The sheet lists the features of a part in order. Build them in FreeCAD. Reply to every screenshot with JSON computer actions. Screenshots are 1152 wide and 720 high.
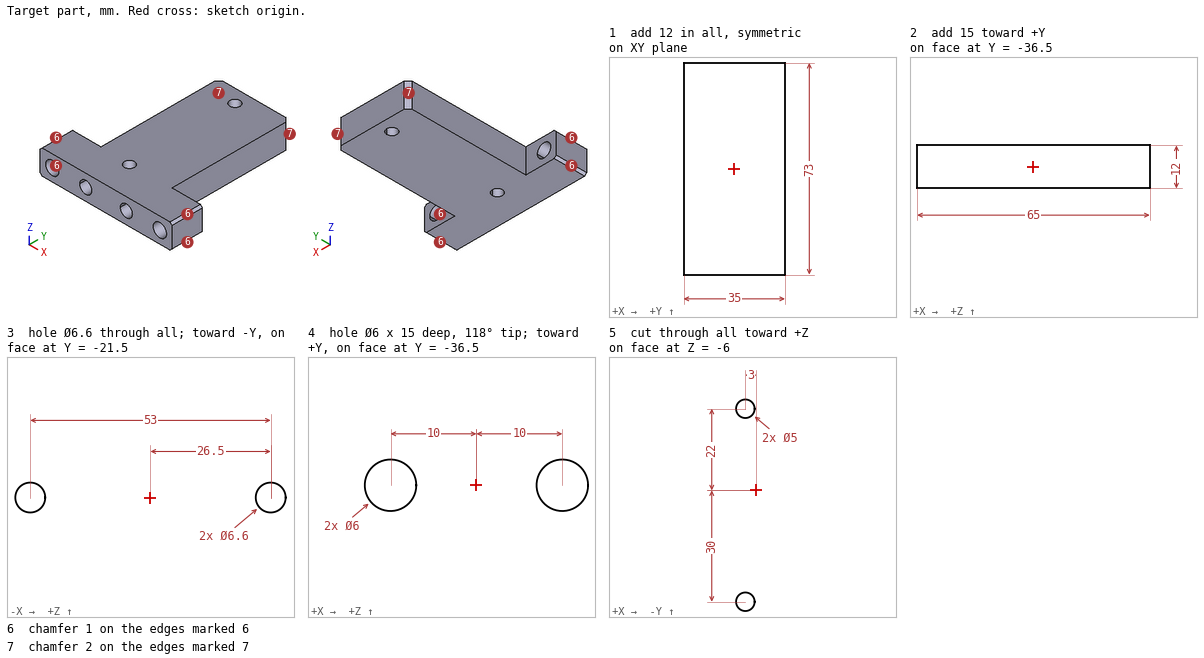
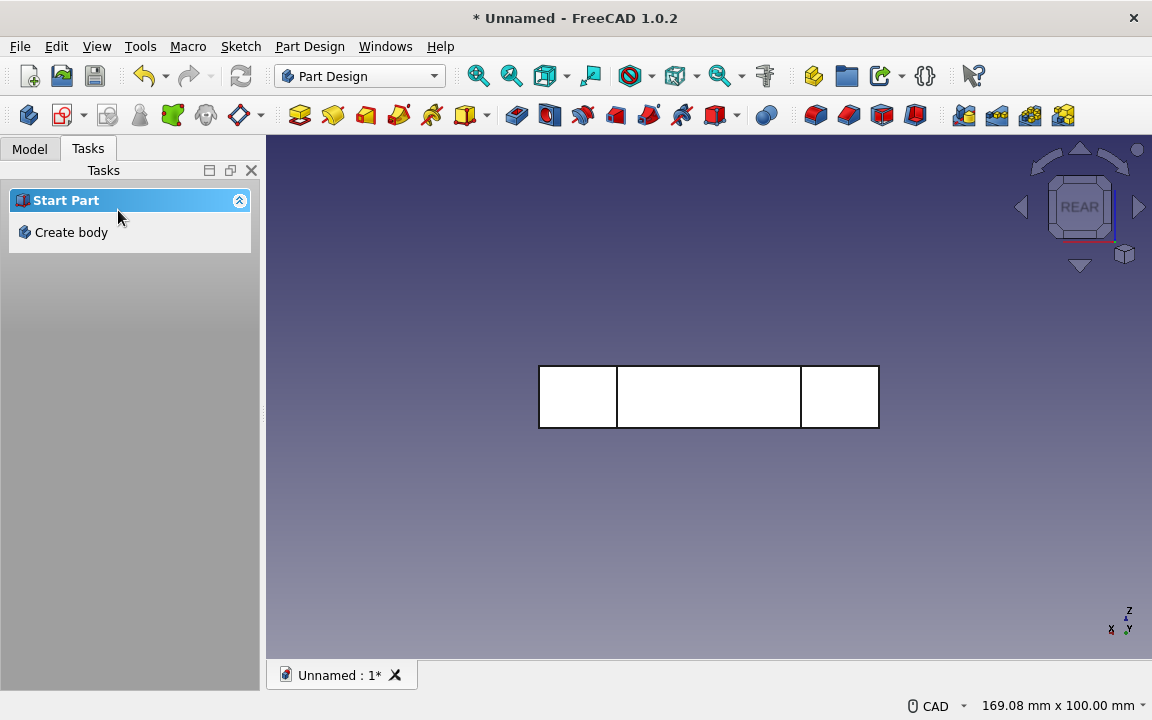
{"action": "left_click", "coordinate": [479, 76]}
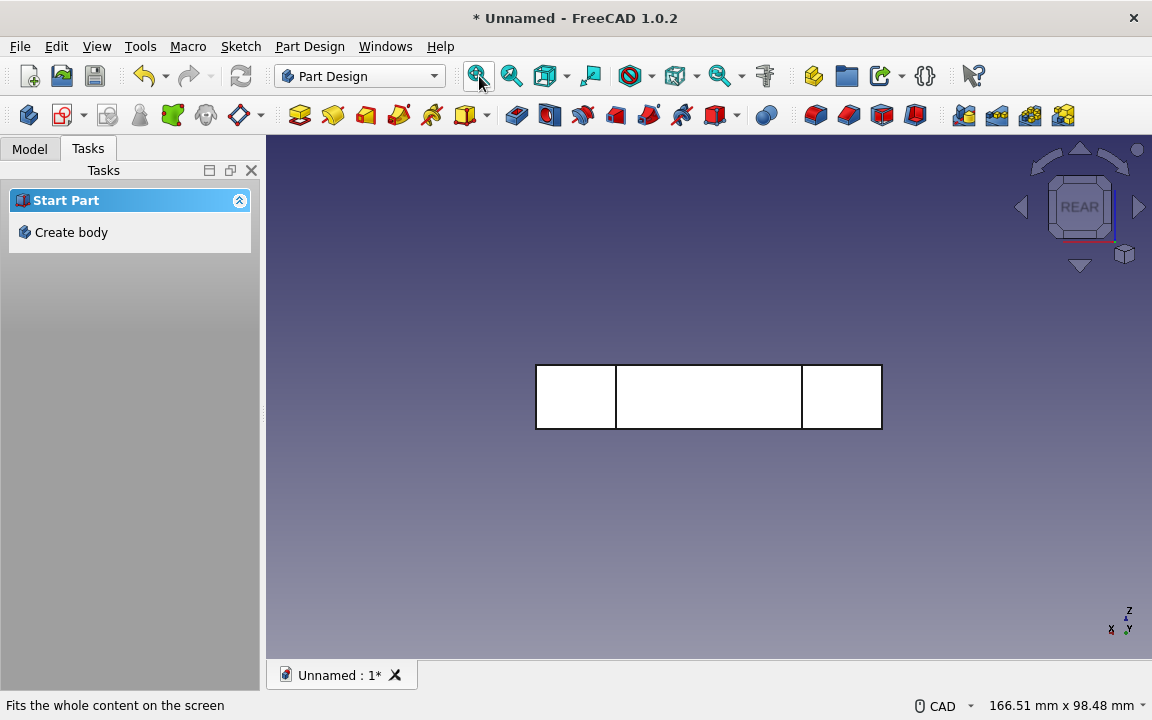
{"action": "left_click", "coordinate": [576, 396]}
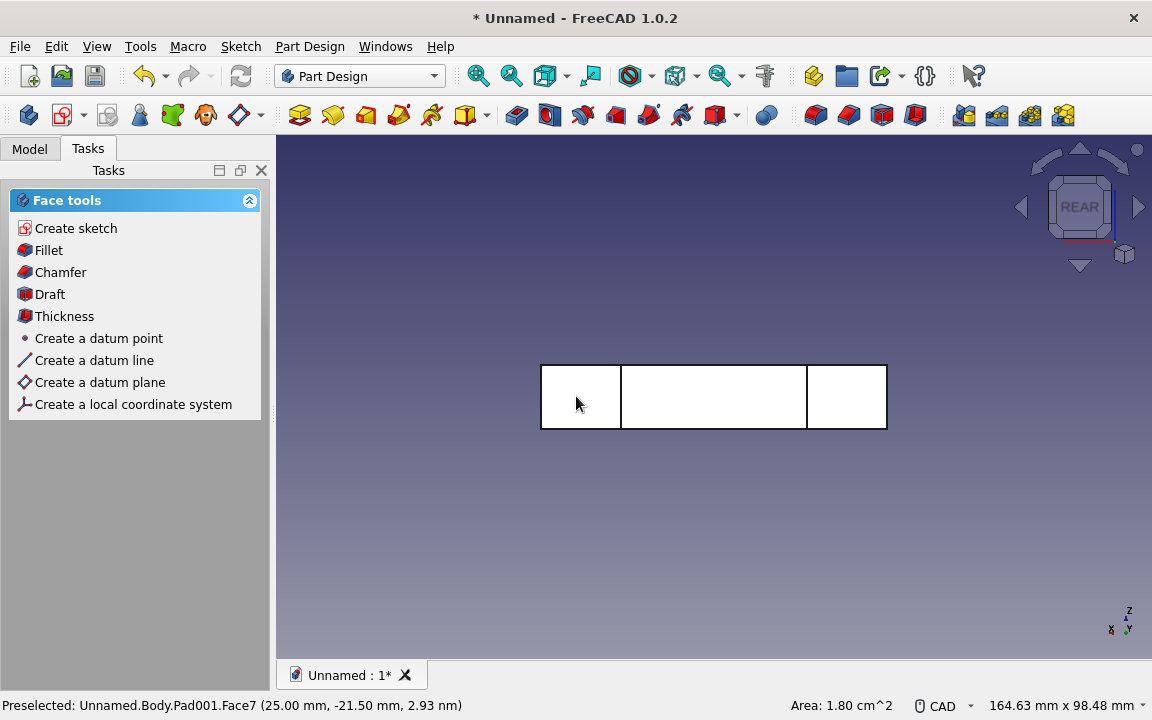
{"action": "left_click", "coordinate": [62, 116]}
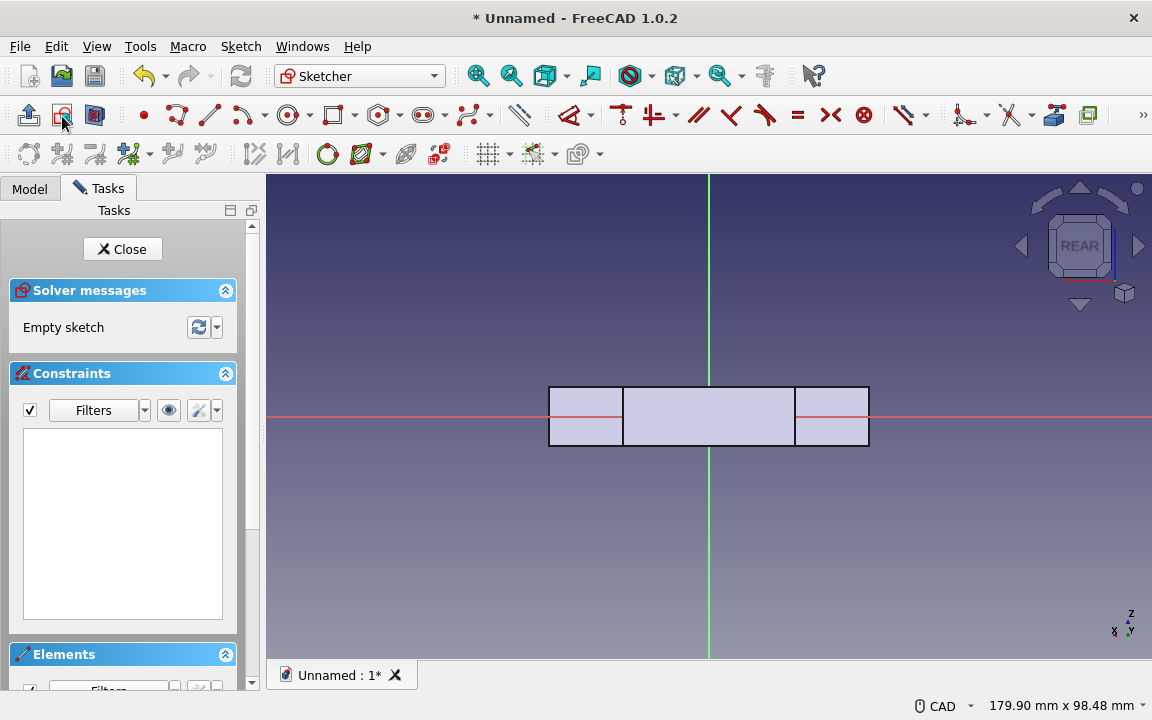
{"action": "scroll", "coordinate": [792, 417], "scroll_direction": "up", "scroll_amount": 3}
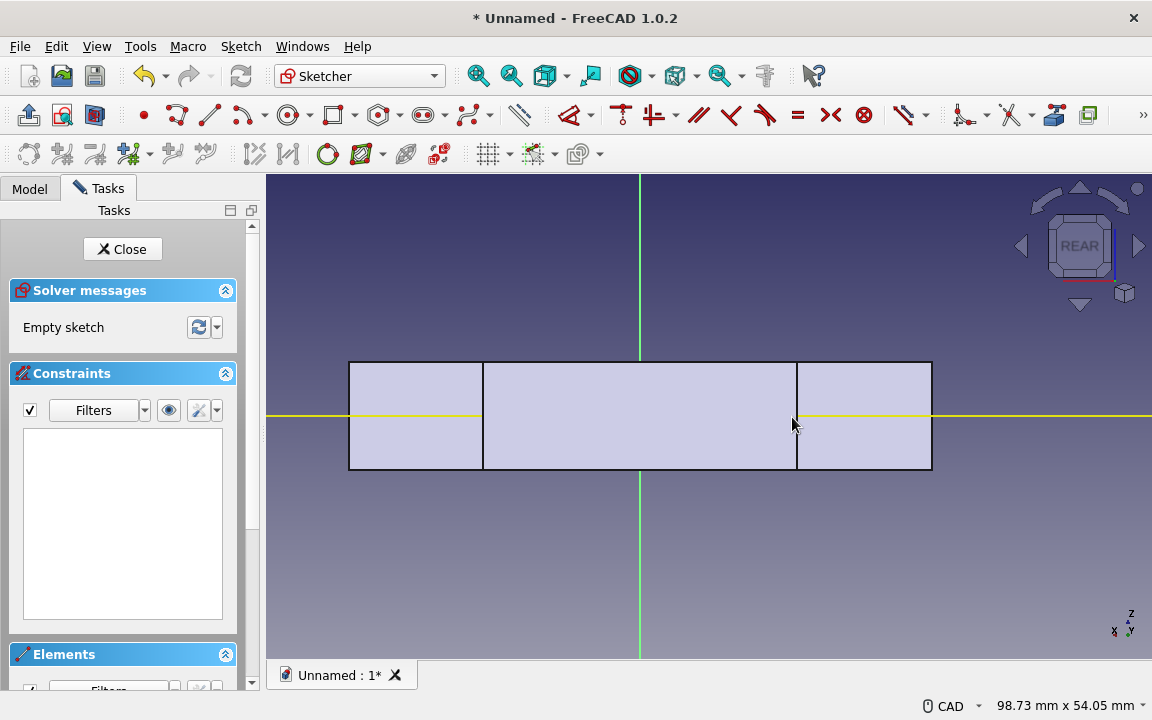
{"action": "left_click", "coordinate": [288, 116]}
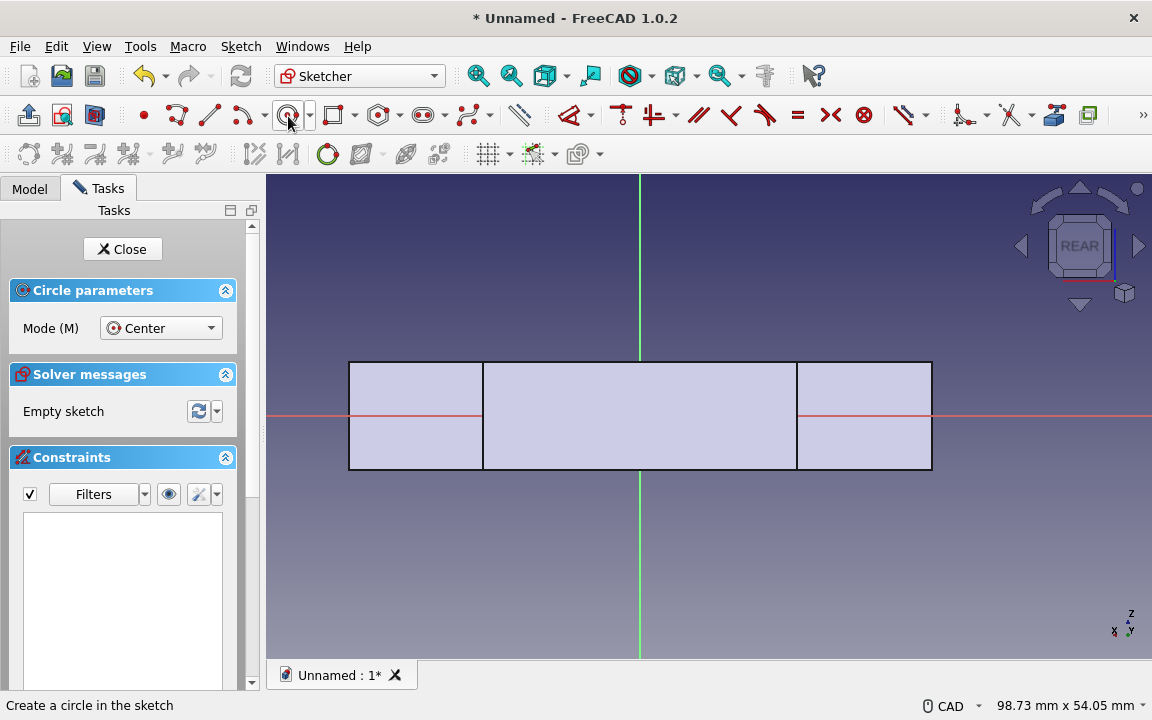
{"action": "left_click", "coordinate": [878, 416]}
{"action": "mouse_move", "coordinate": [899, 395]}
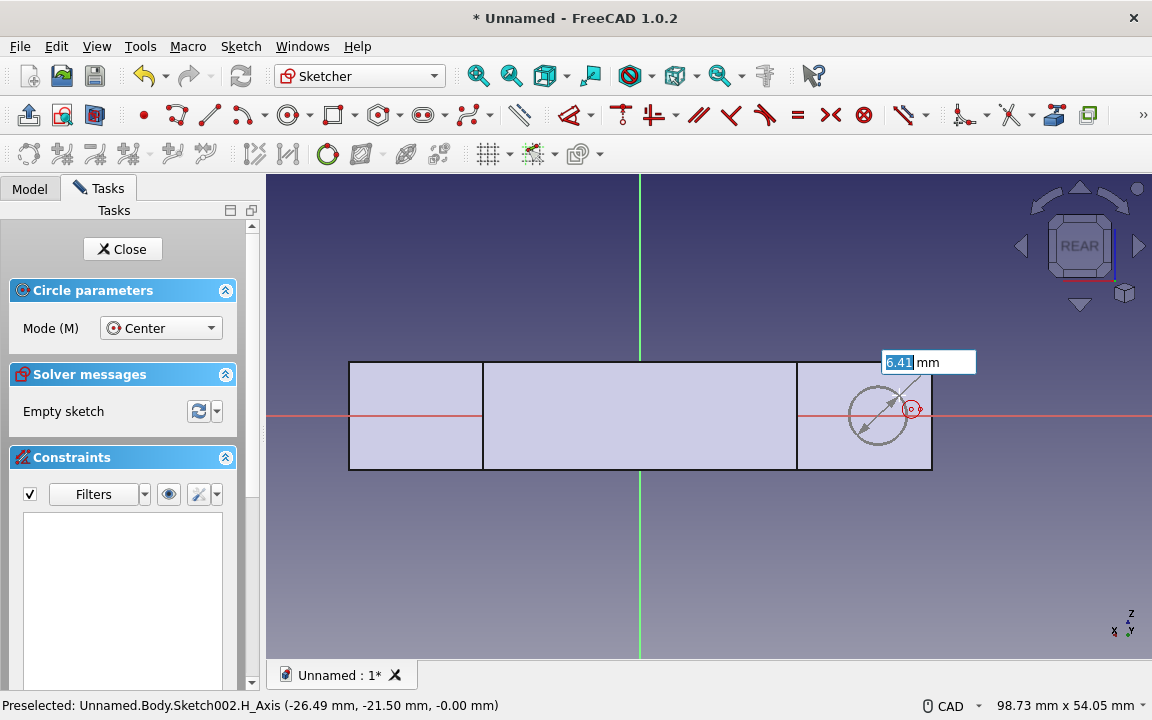
{"action": "type", "text": "6.6"}
{"action": "key", "text": "Return"}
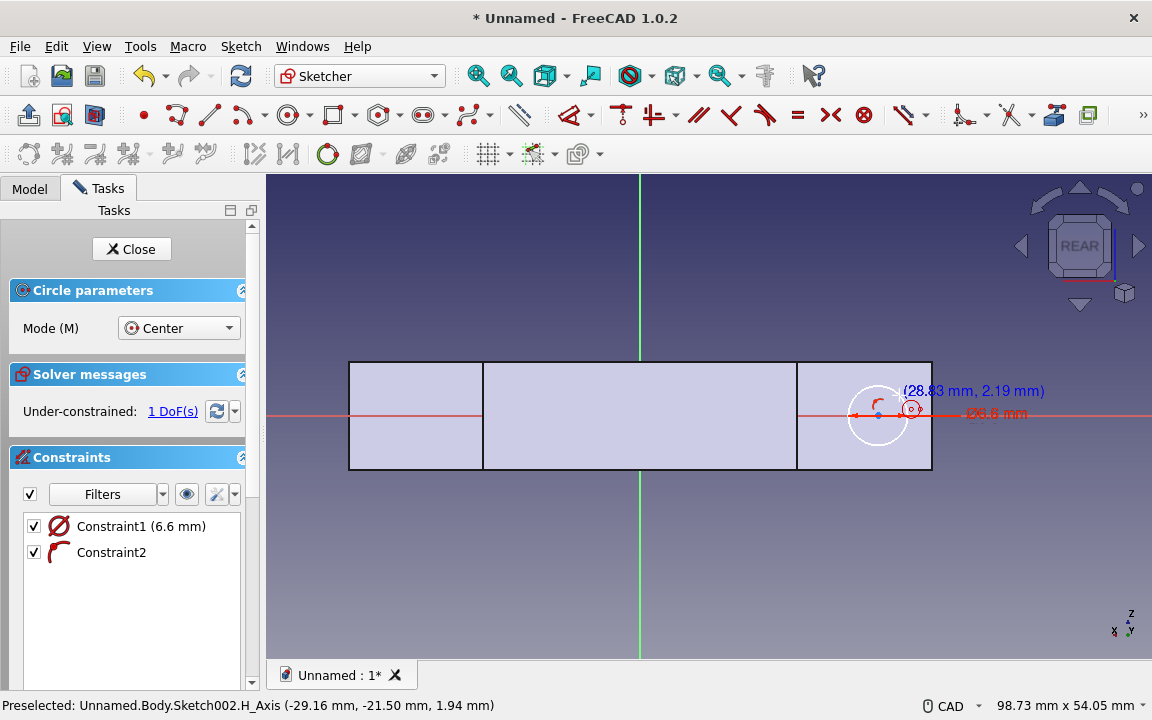
{"action": "left_click", "coordinate": [402, 416]}
{"action": "mouse_move", "coordinate": [423, 395]}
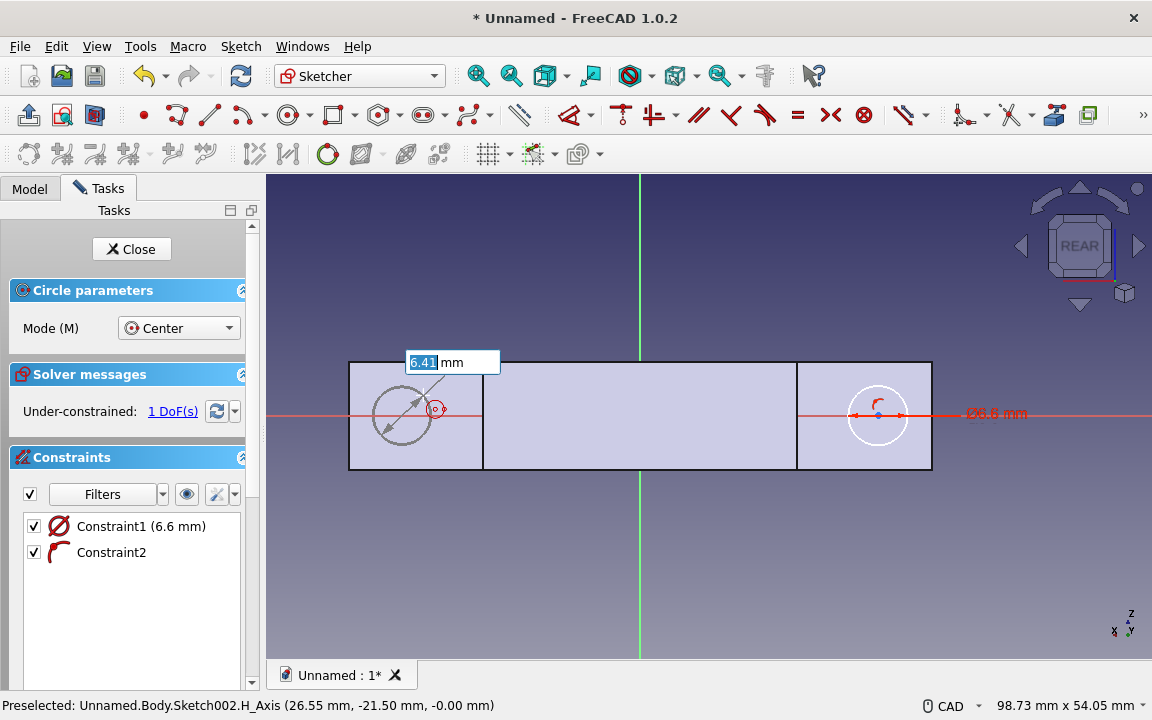
{"action": "type", "text": "6.6"}
{"action": "key", "text": "Return"}
{"action": "key", "text": "Escape"}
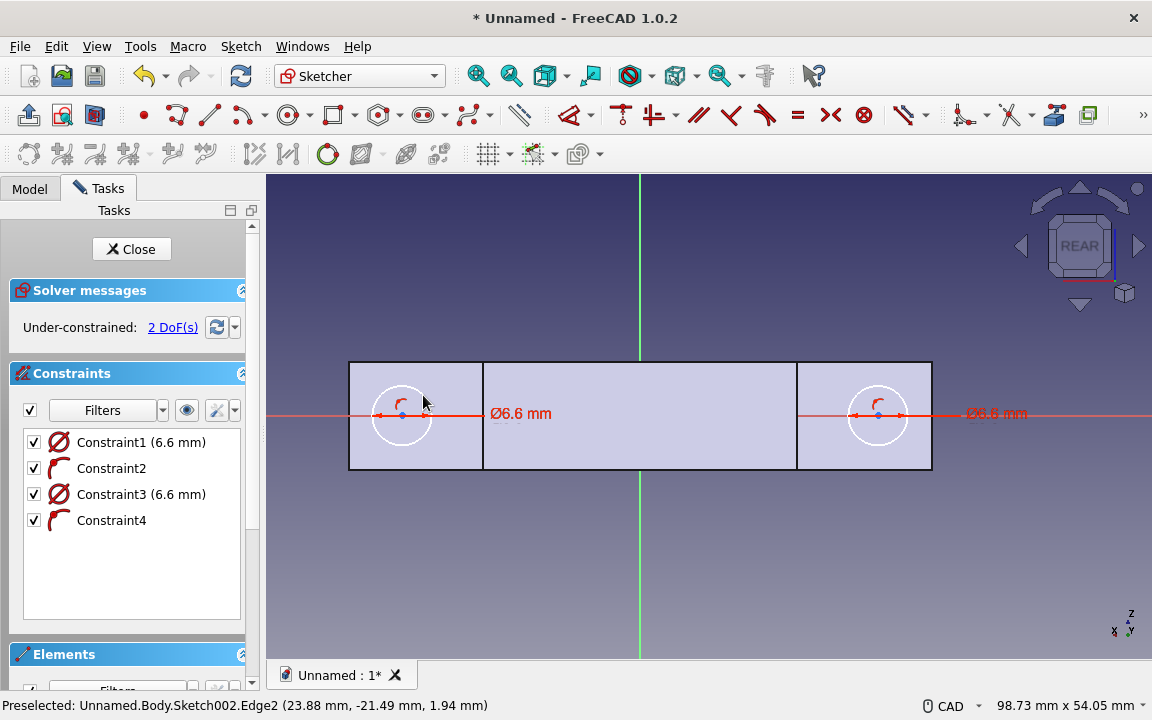
{"action": "left_click", "coordinate": [878, 416]}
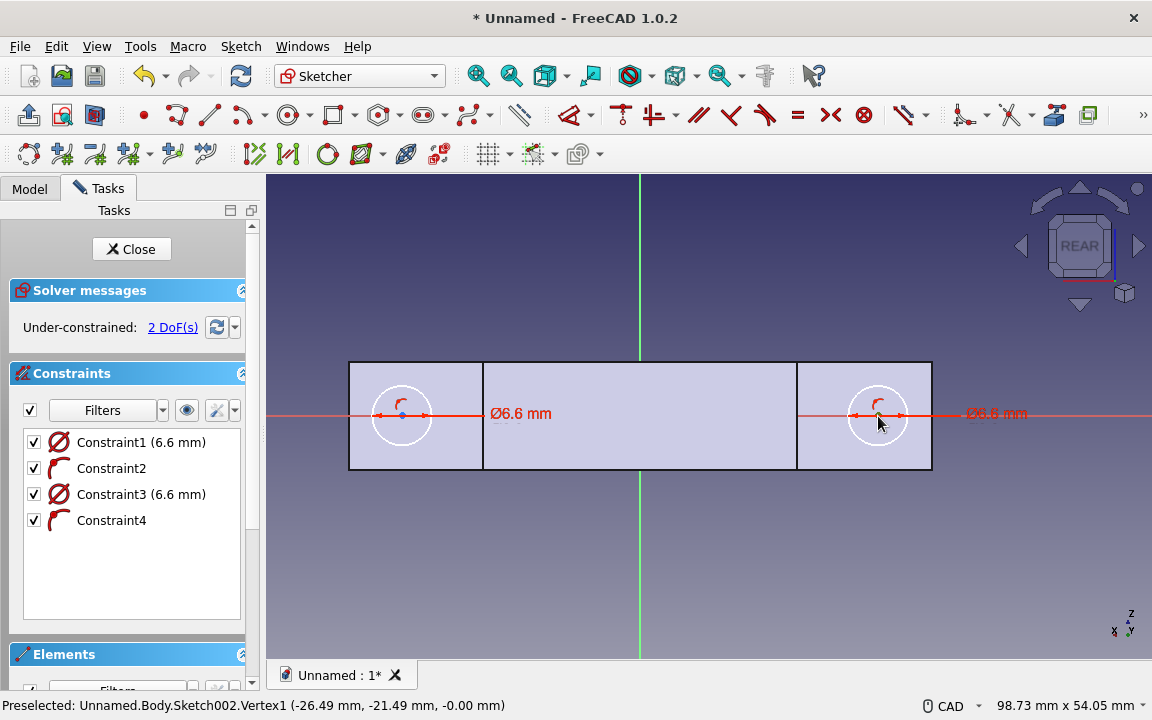
{"action": "left_click", "coordinate": [402, 416]}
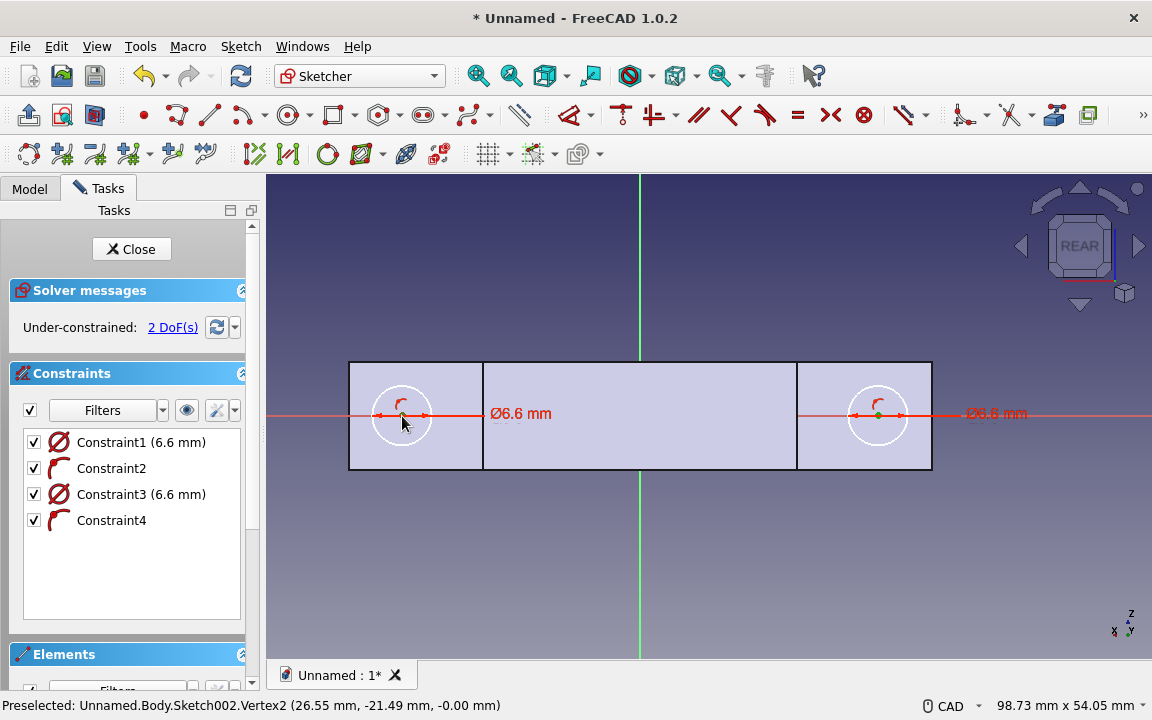
{"action": "left_click", "coordinate": [590, 116]}